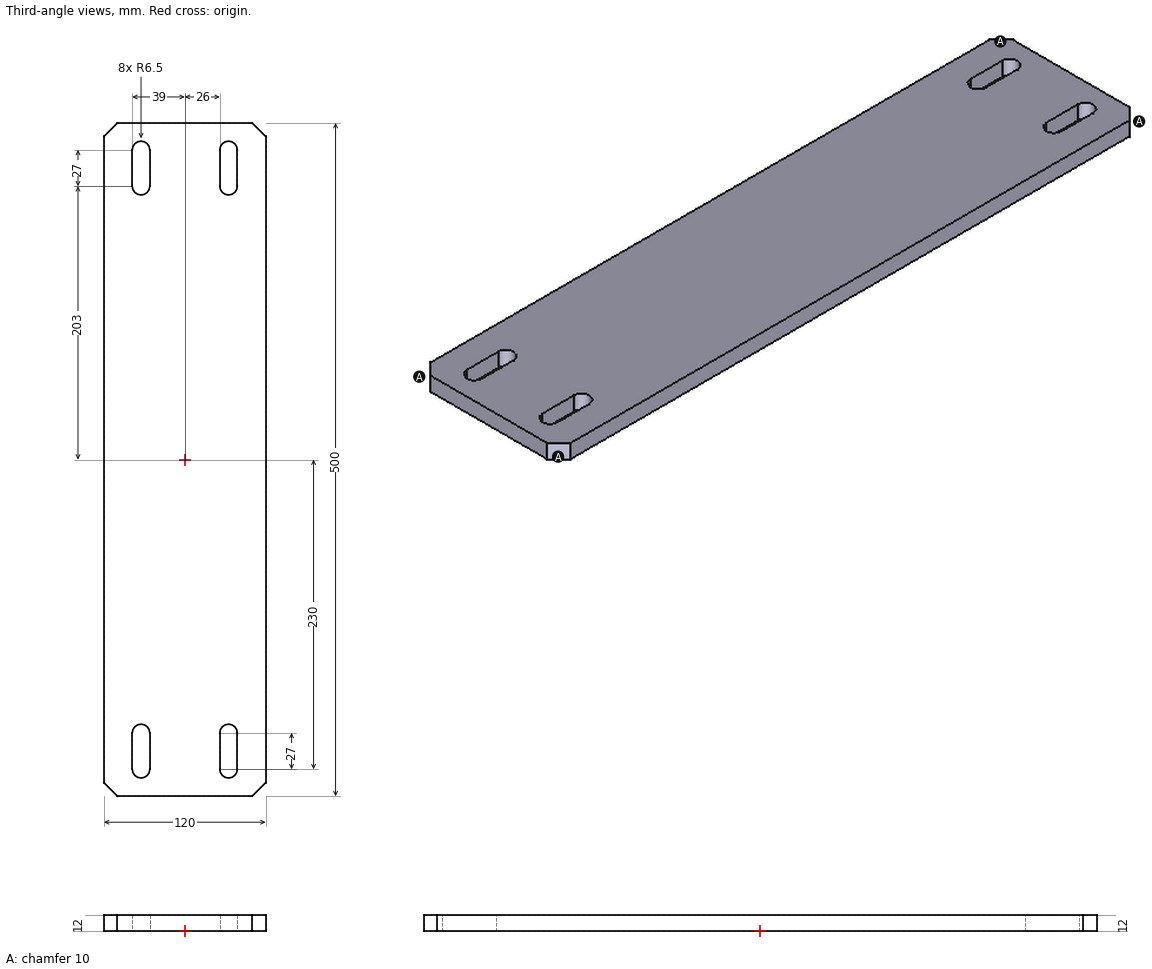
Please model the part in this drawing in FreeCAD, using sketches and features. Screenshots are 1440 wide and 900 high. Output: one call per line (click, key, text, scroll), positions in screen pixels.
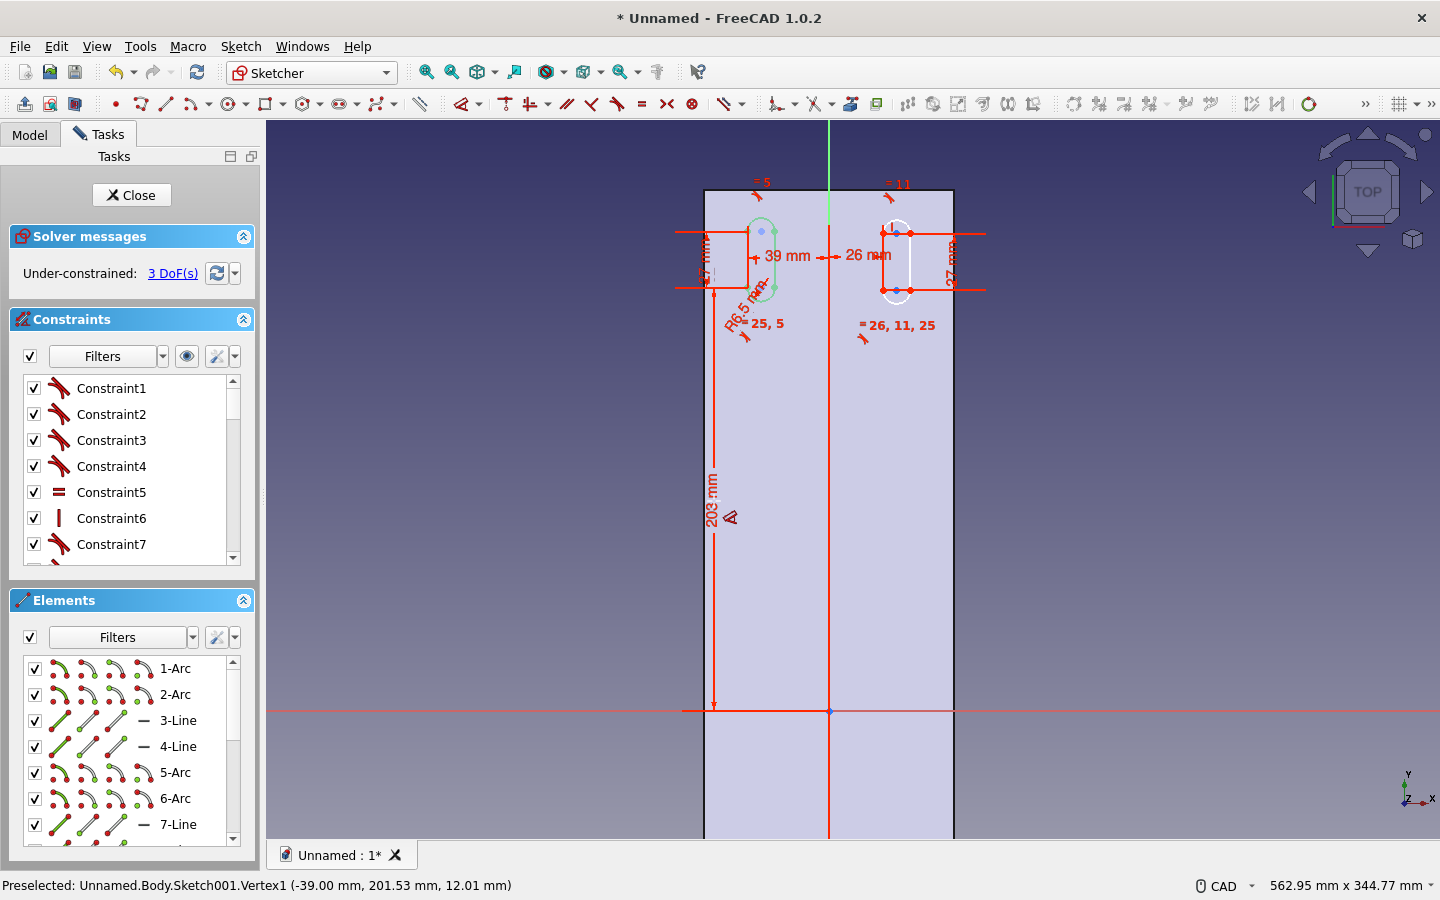
click(883, 290)
click(917, 501)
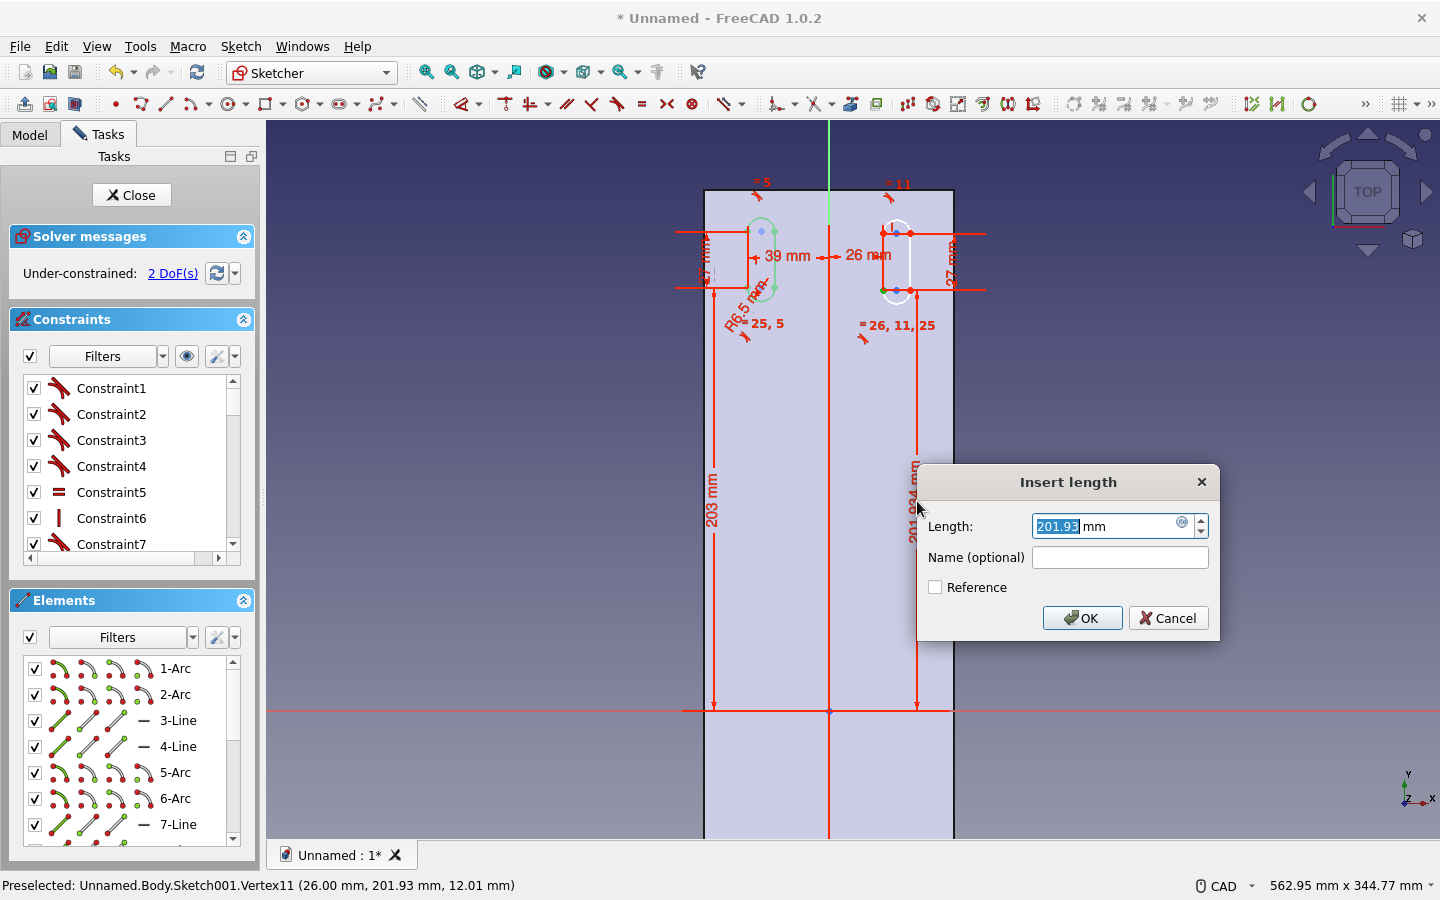
text(203)
key(Return)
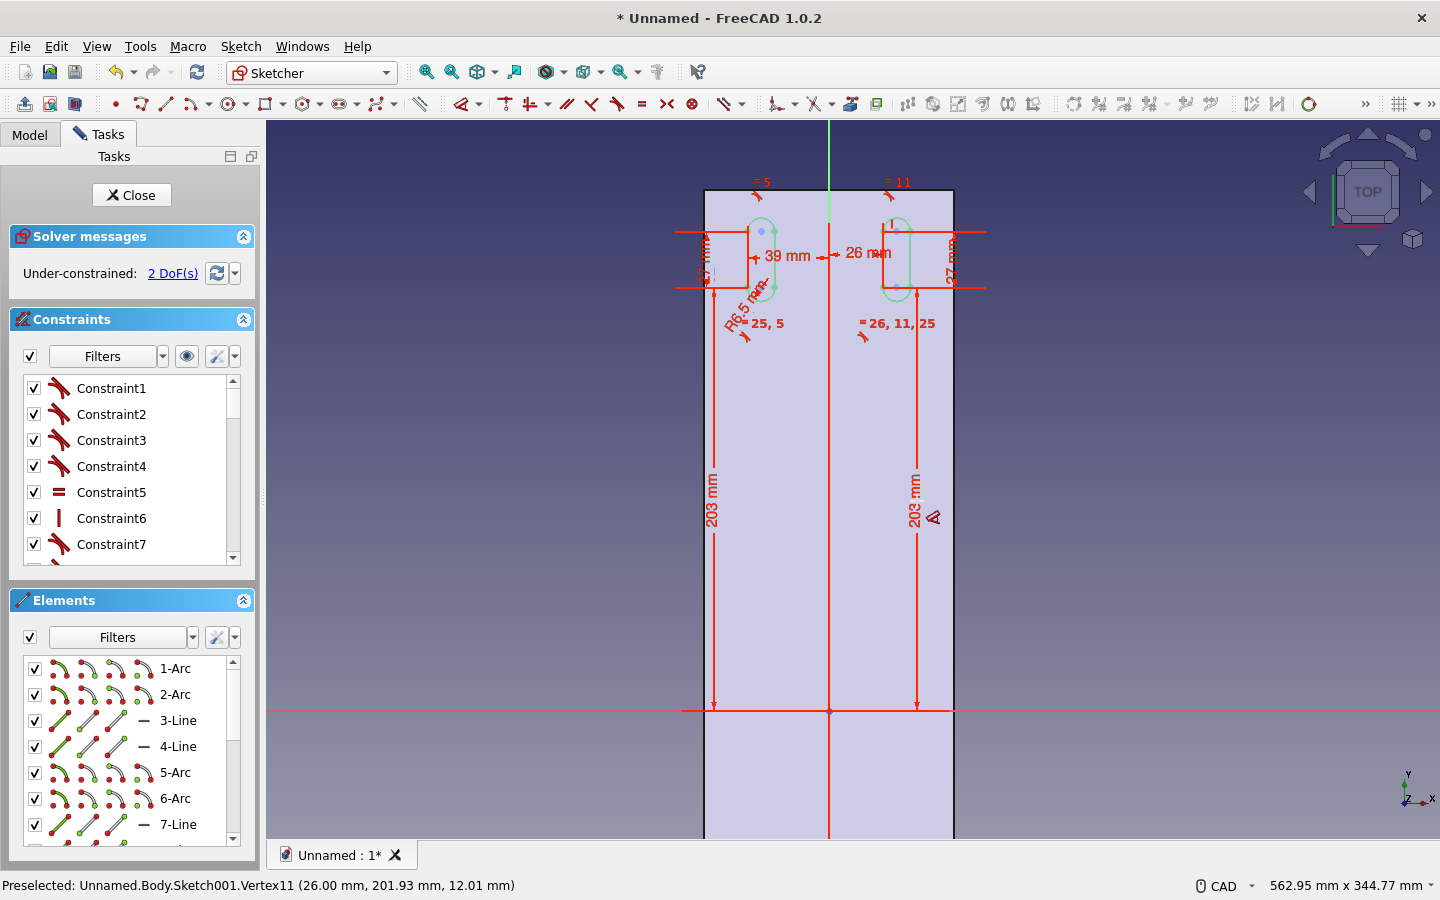
scroll(748, 290, down, 4)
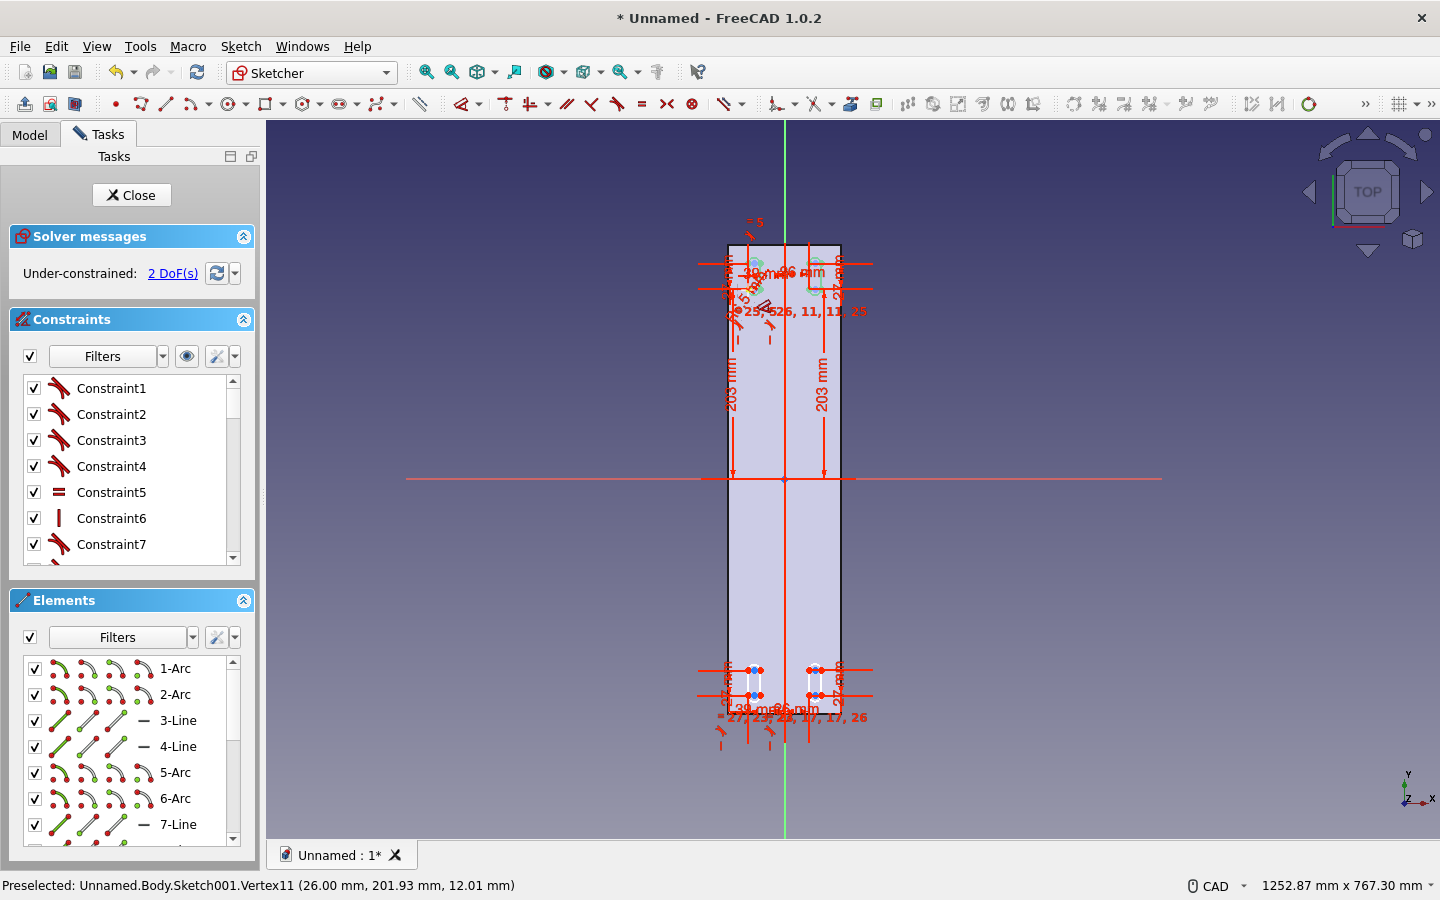
scroll(809, 696, up, 4)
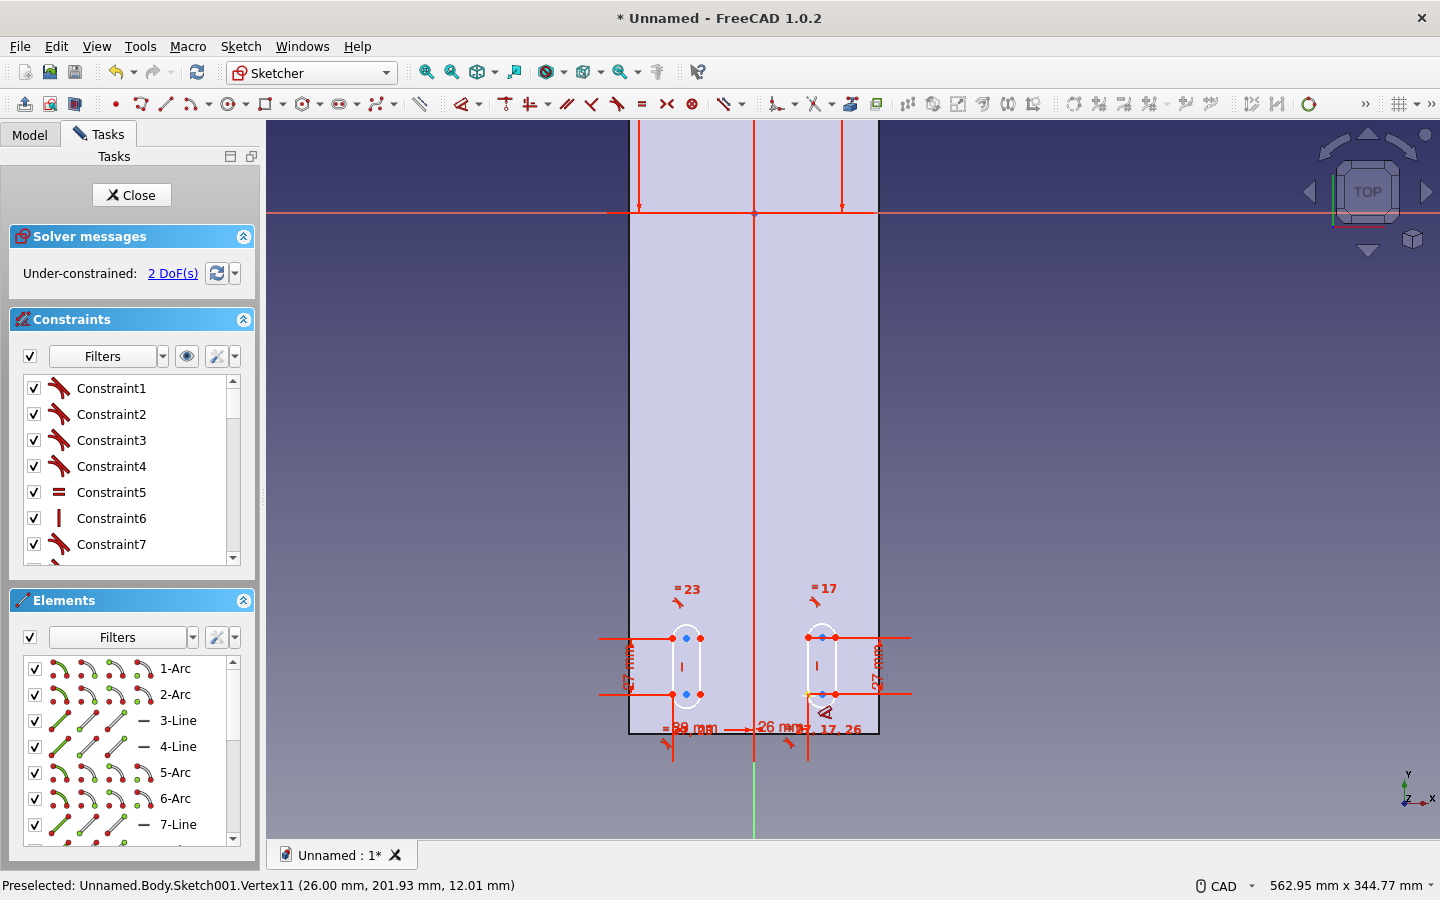
click(808, 694)
click(842, 454)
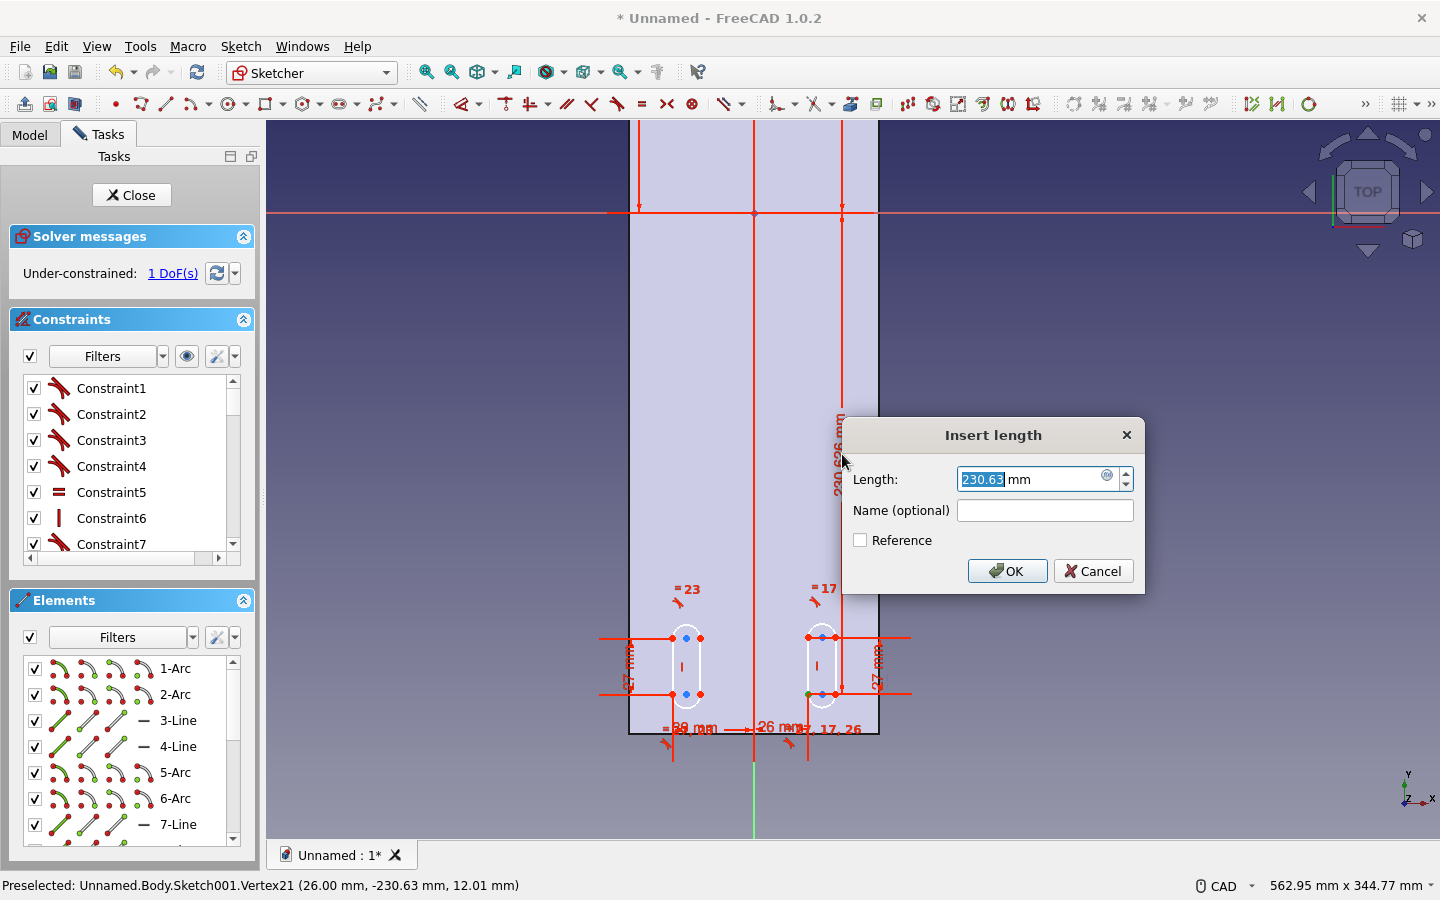
text(230)
key(Return)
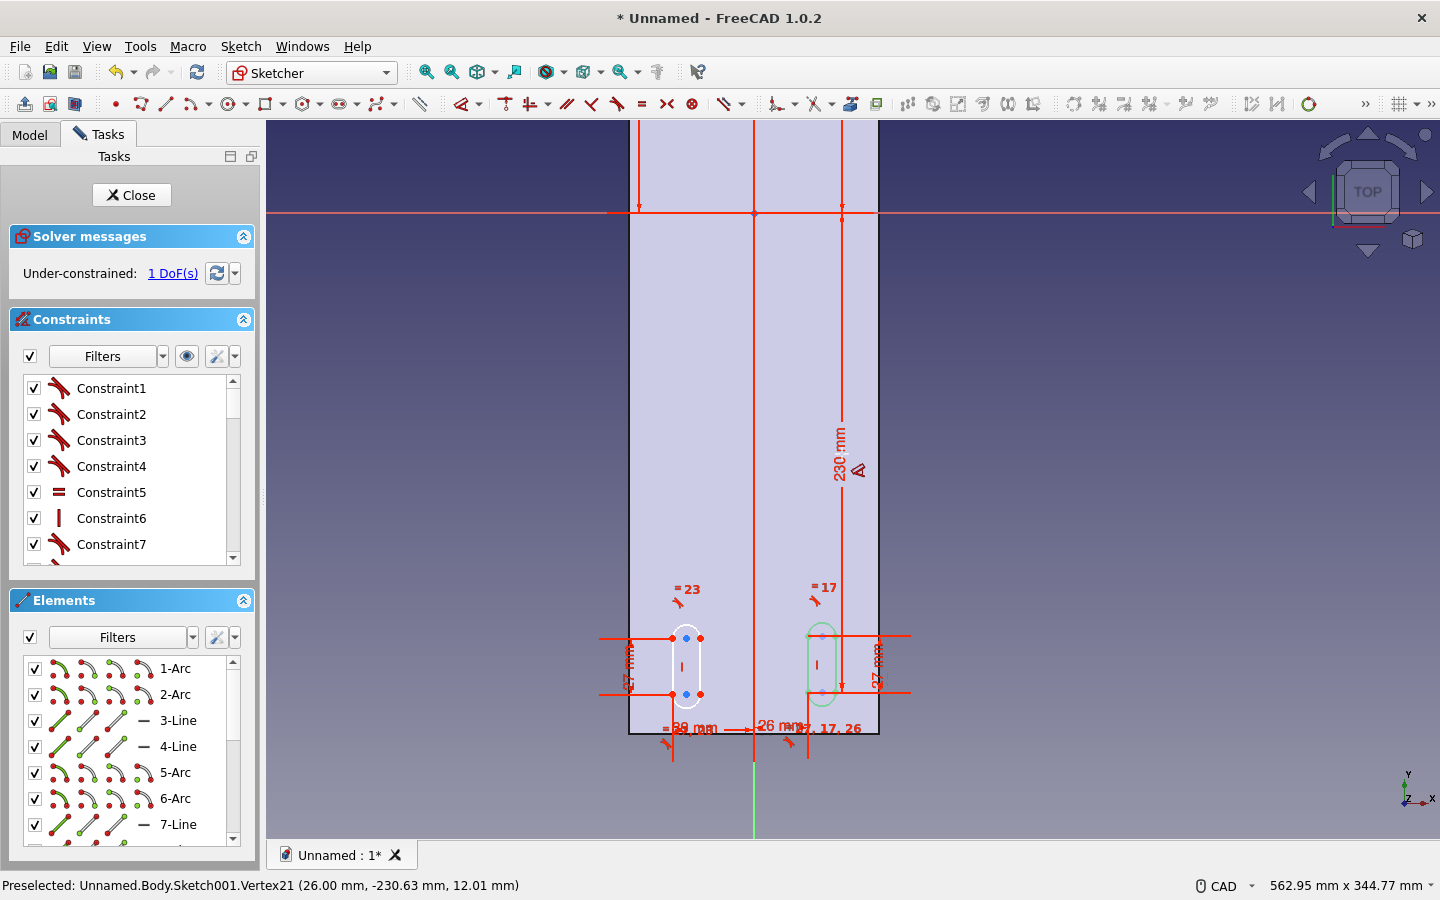
click(673, 695)
click(639, 454)